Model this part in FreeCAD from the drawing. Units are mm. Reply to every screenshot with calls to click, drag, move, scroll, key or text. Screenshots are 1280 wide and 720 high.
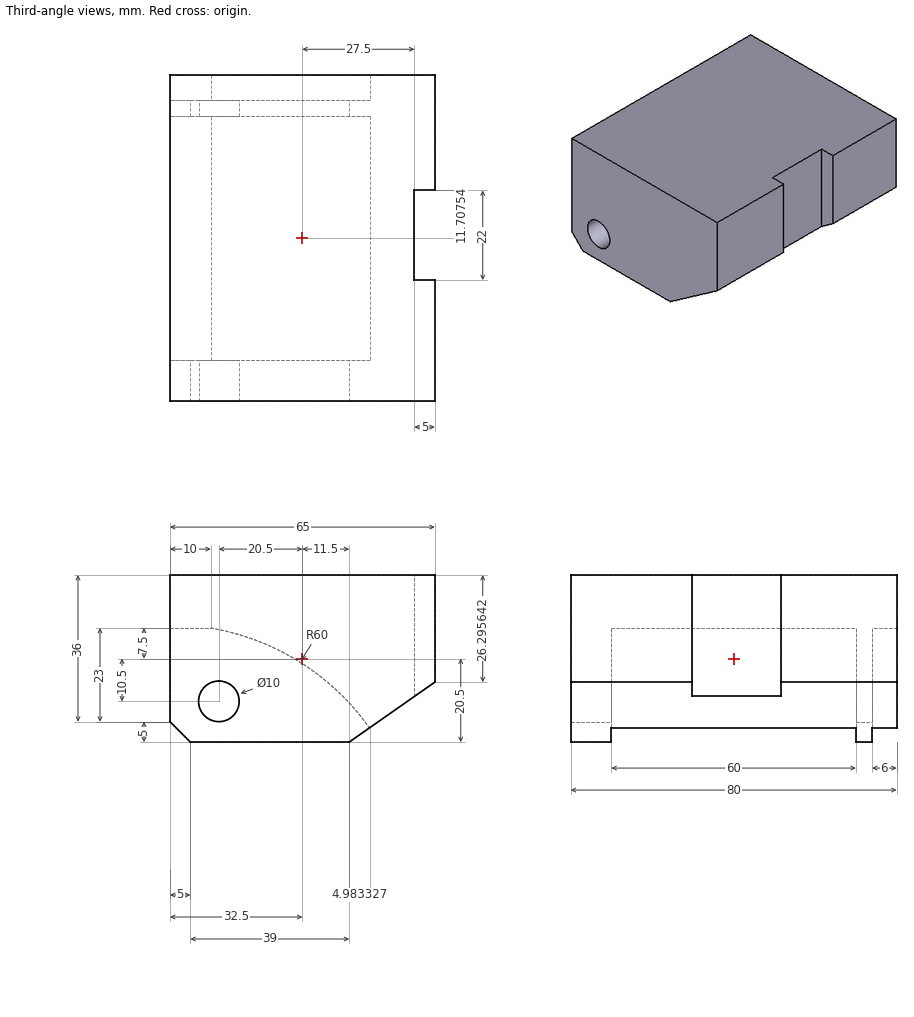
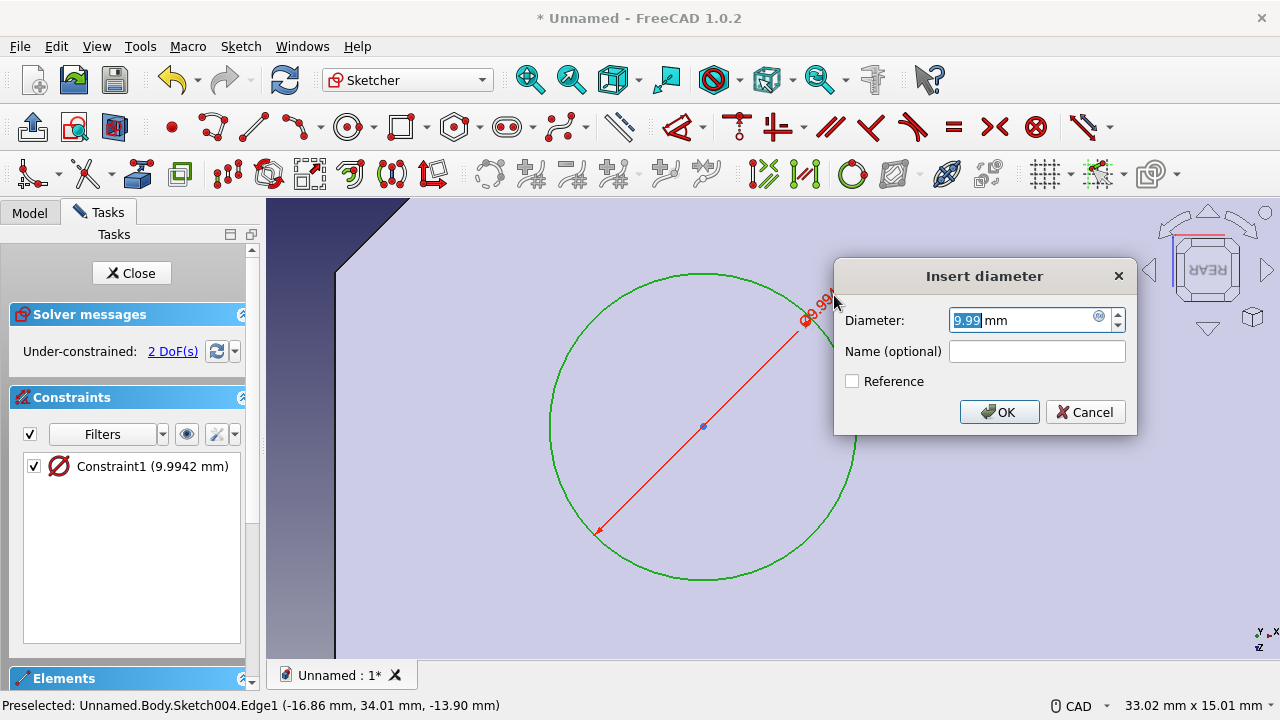
text(10)
key(Return)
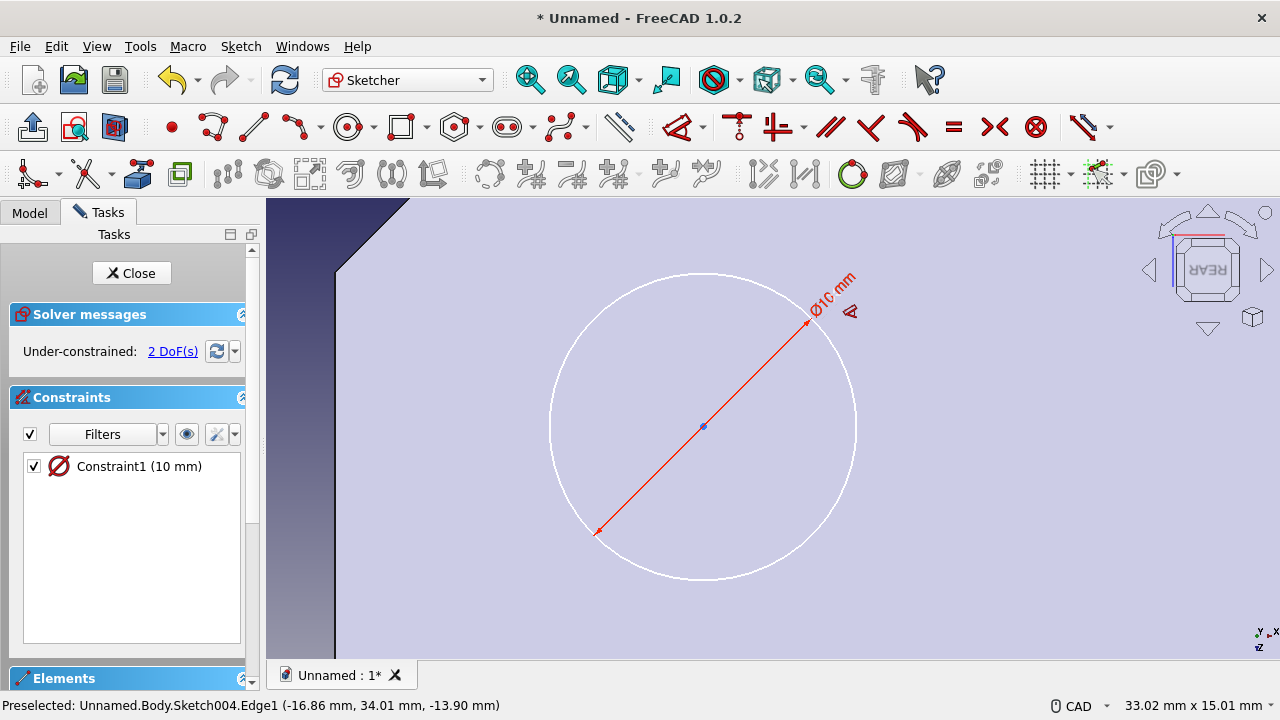
click(703, 427)
click(909, 393)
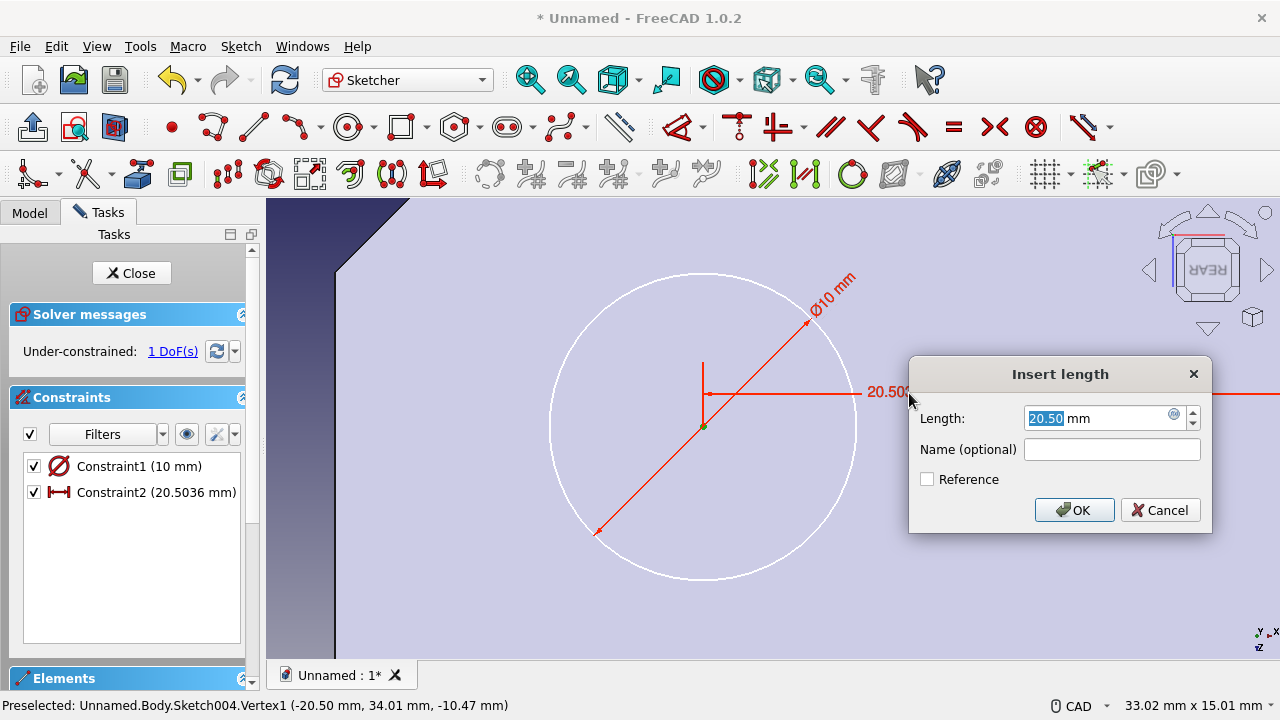
text(20.5)
key(Return)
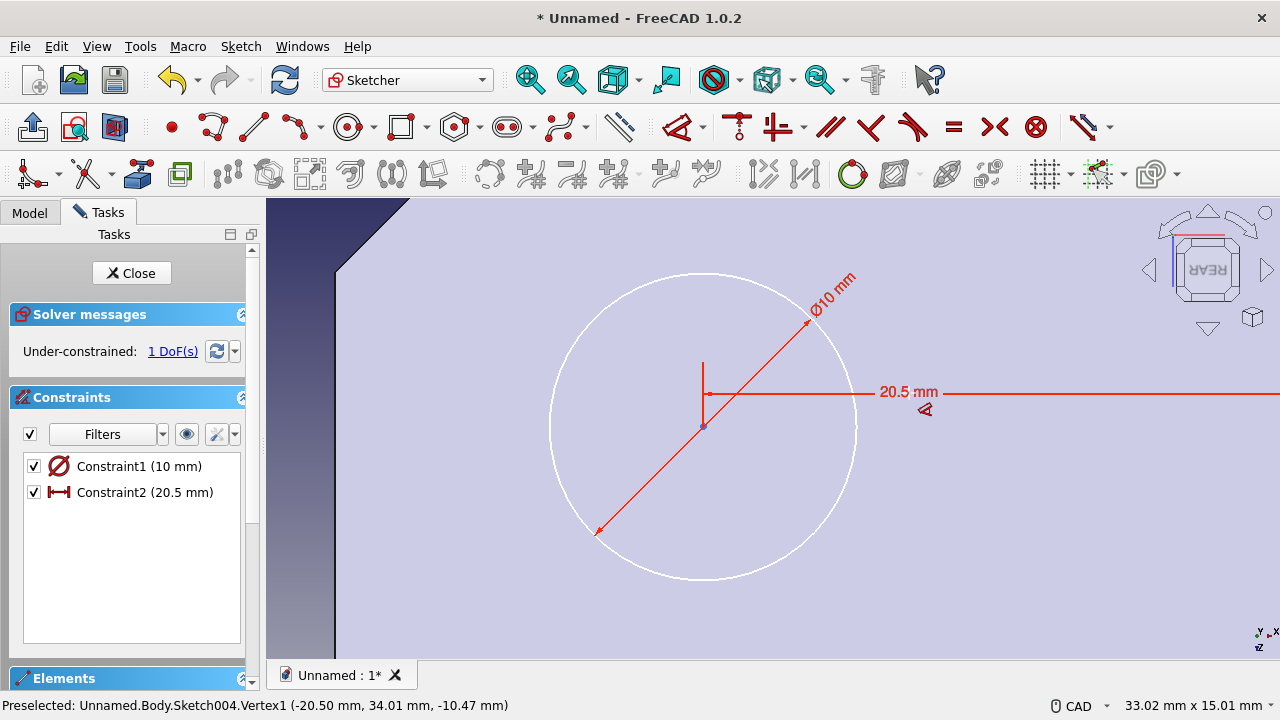
click(703, 427)
click(669, 529)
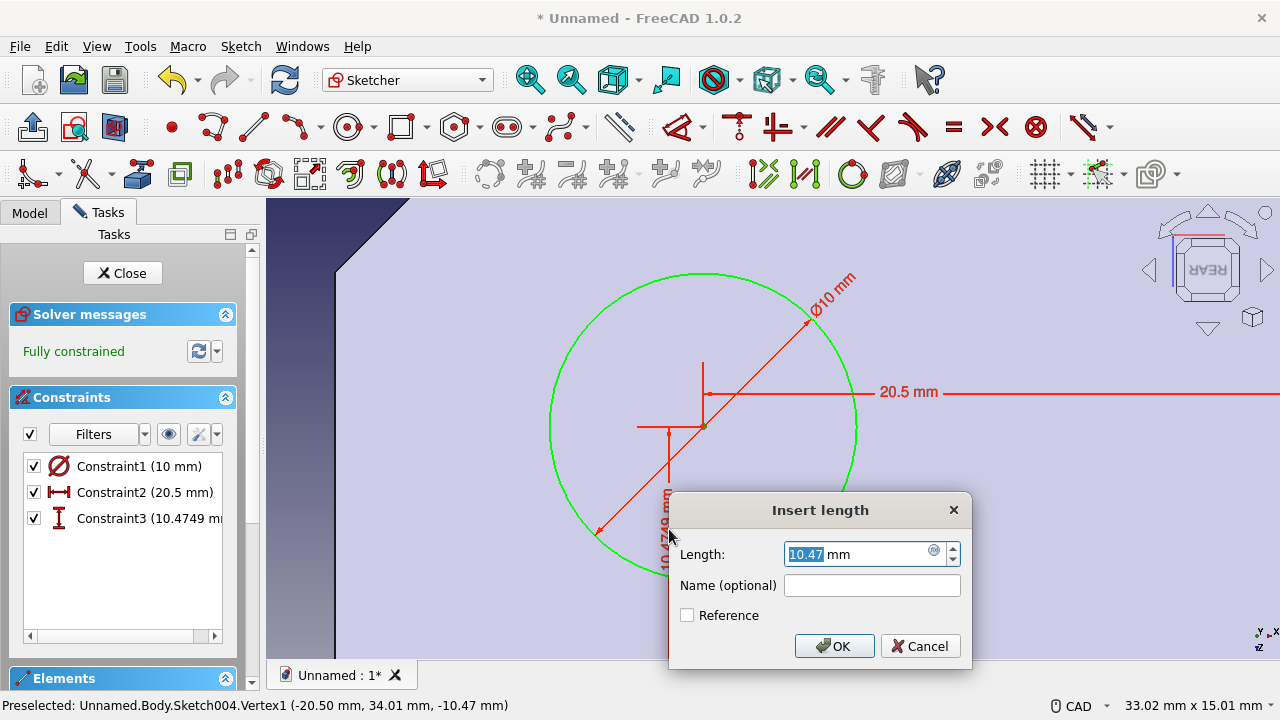
text(10.5)
key(Return)
key(Escape)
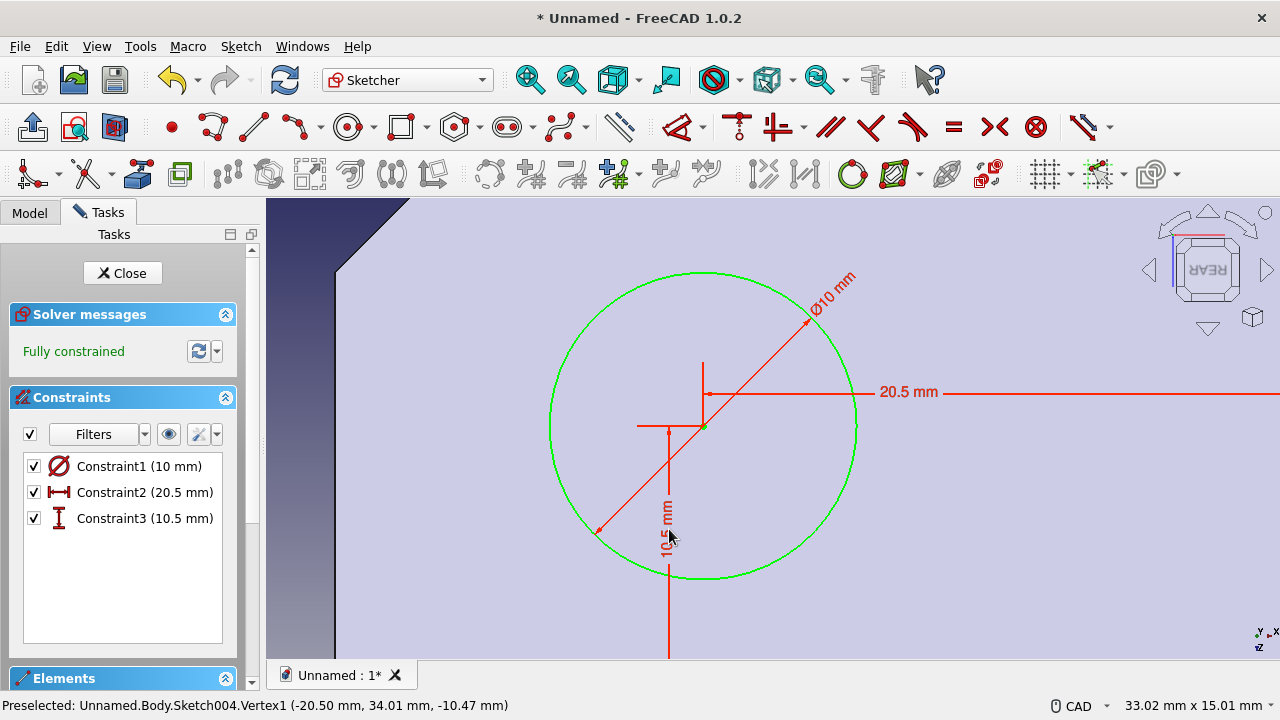
click(123, 273)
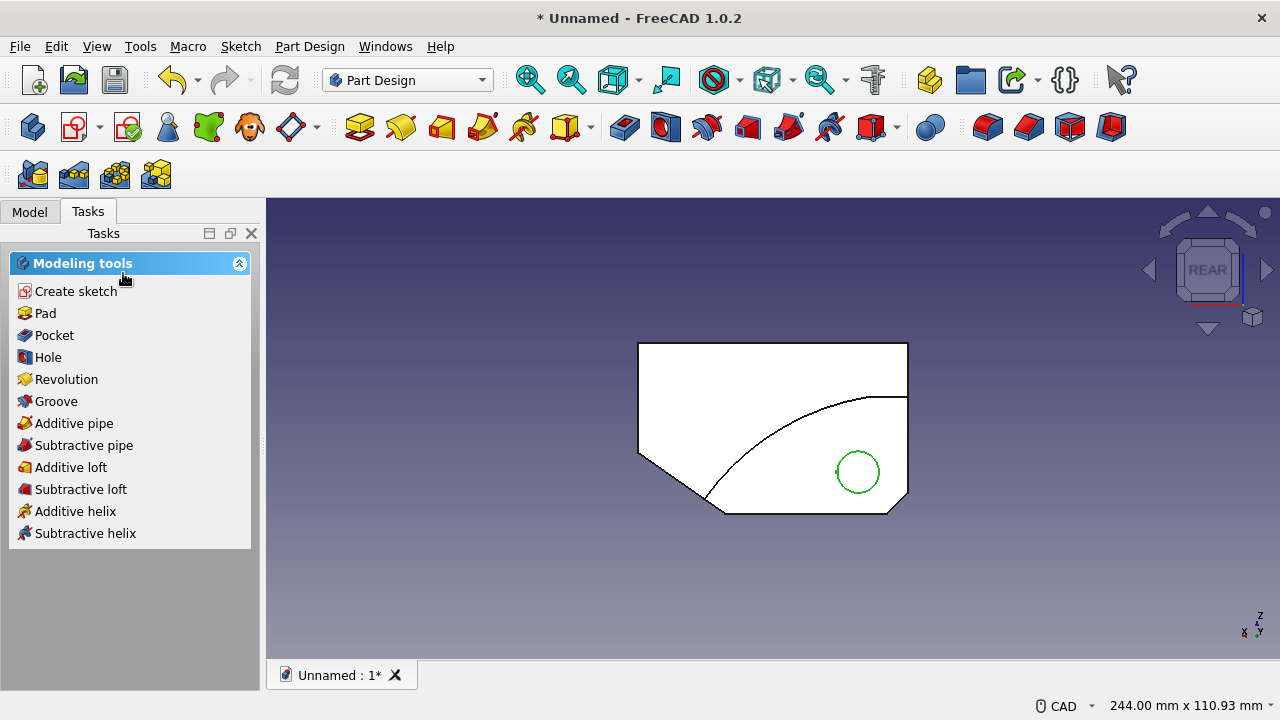
click(625, 128)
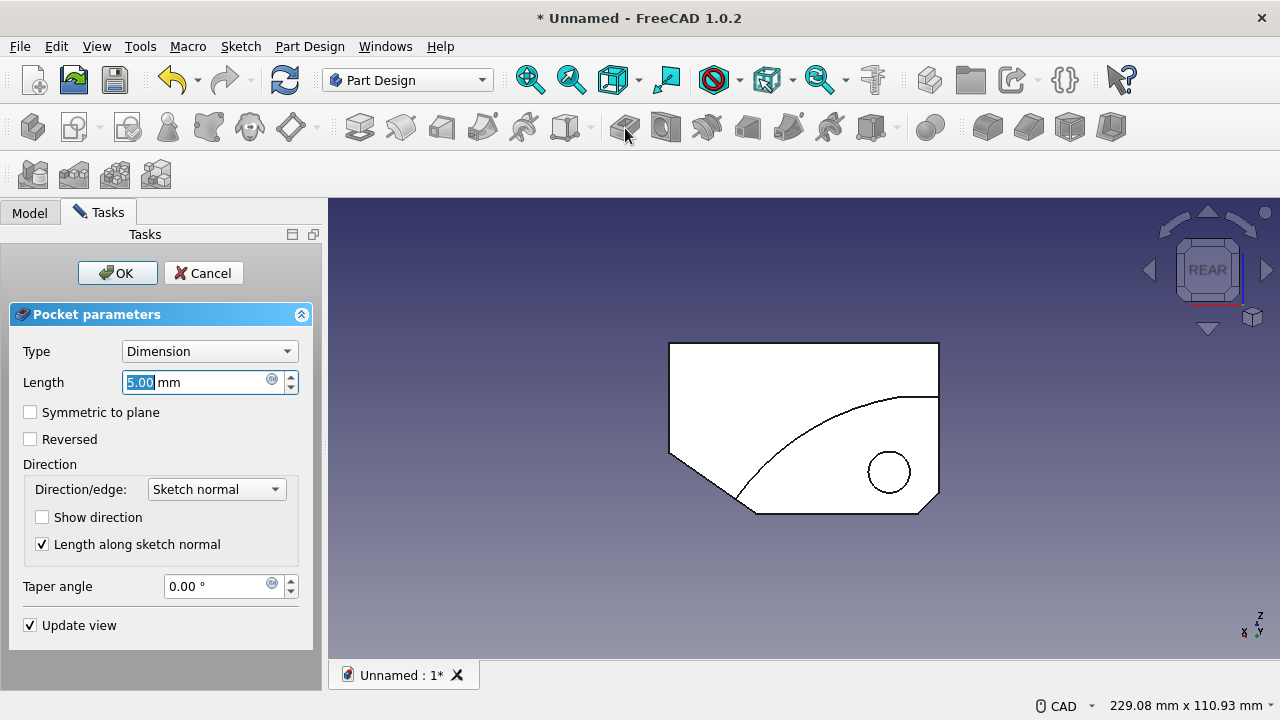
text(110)
key(Tab)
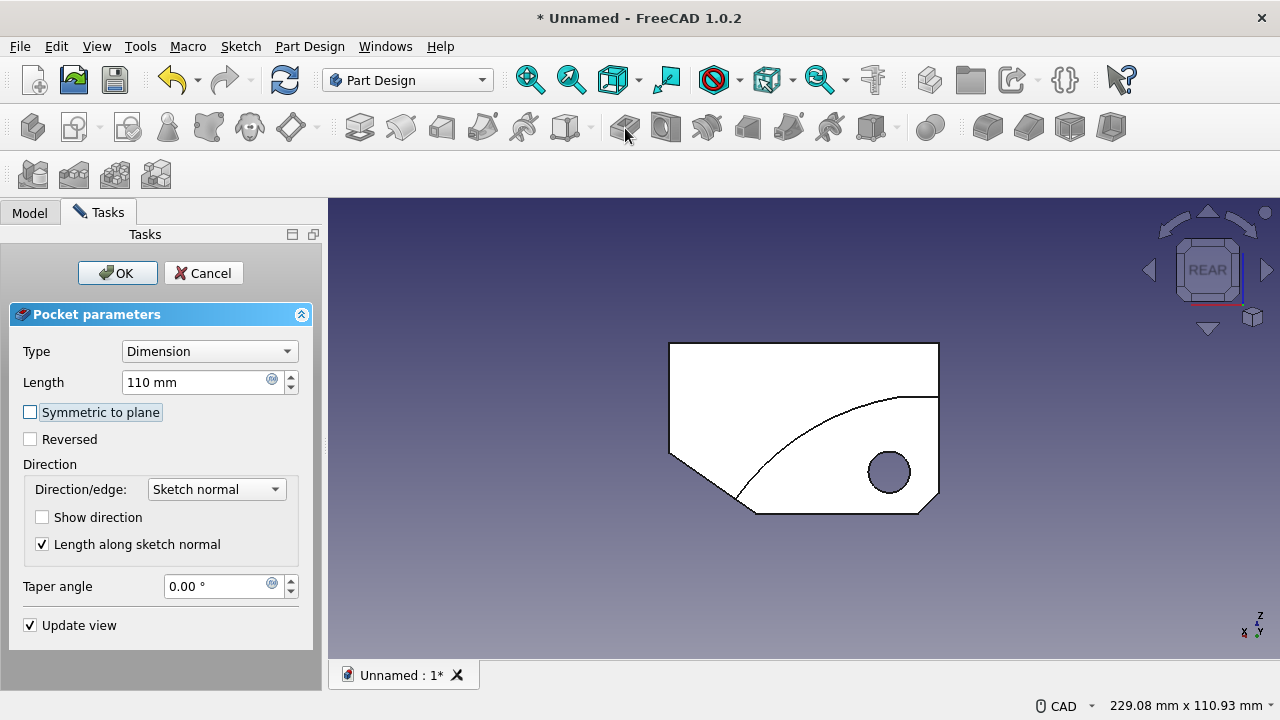
click(118, 273)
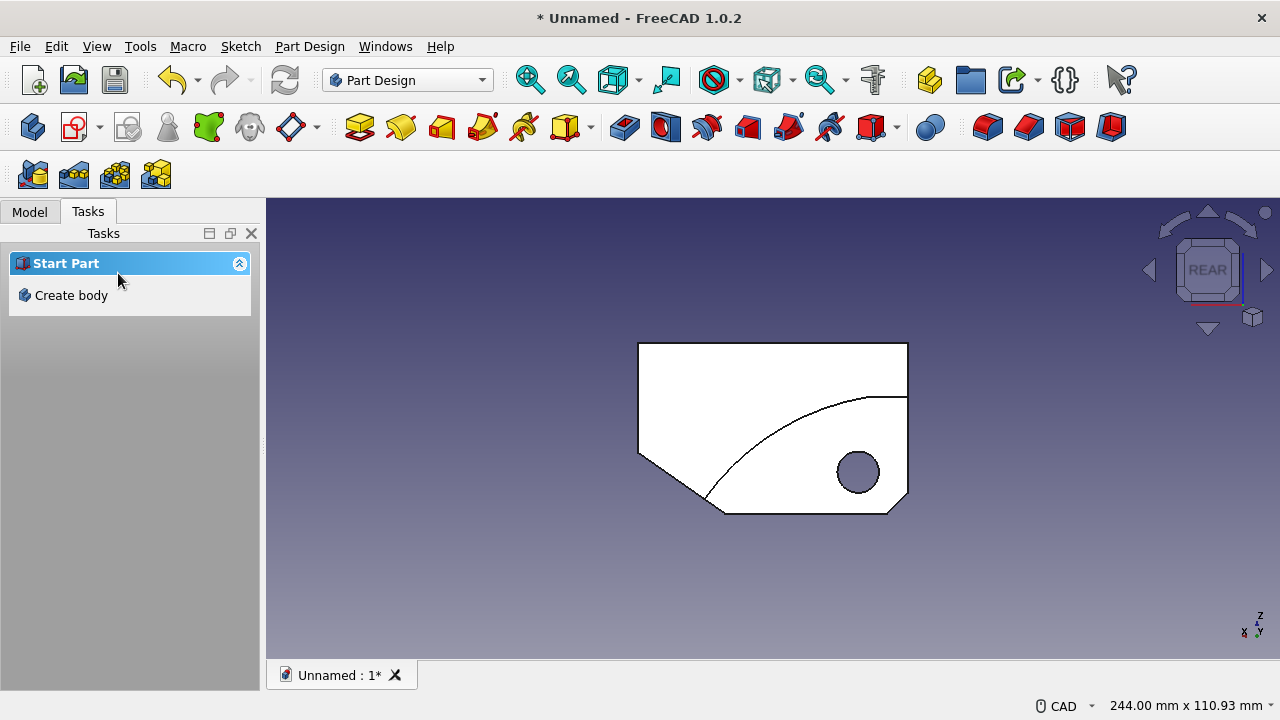
key(0)